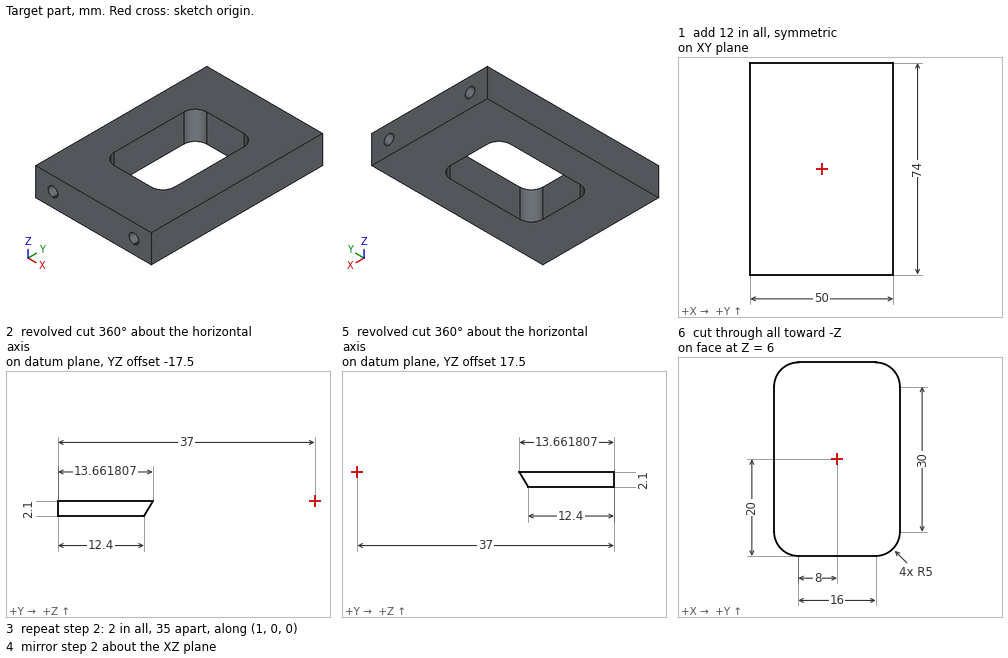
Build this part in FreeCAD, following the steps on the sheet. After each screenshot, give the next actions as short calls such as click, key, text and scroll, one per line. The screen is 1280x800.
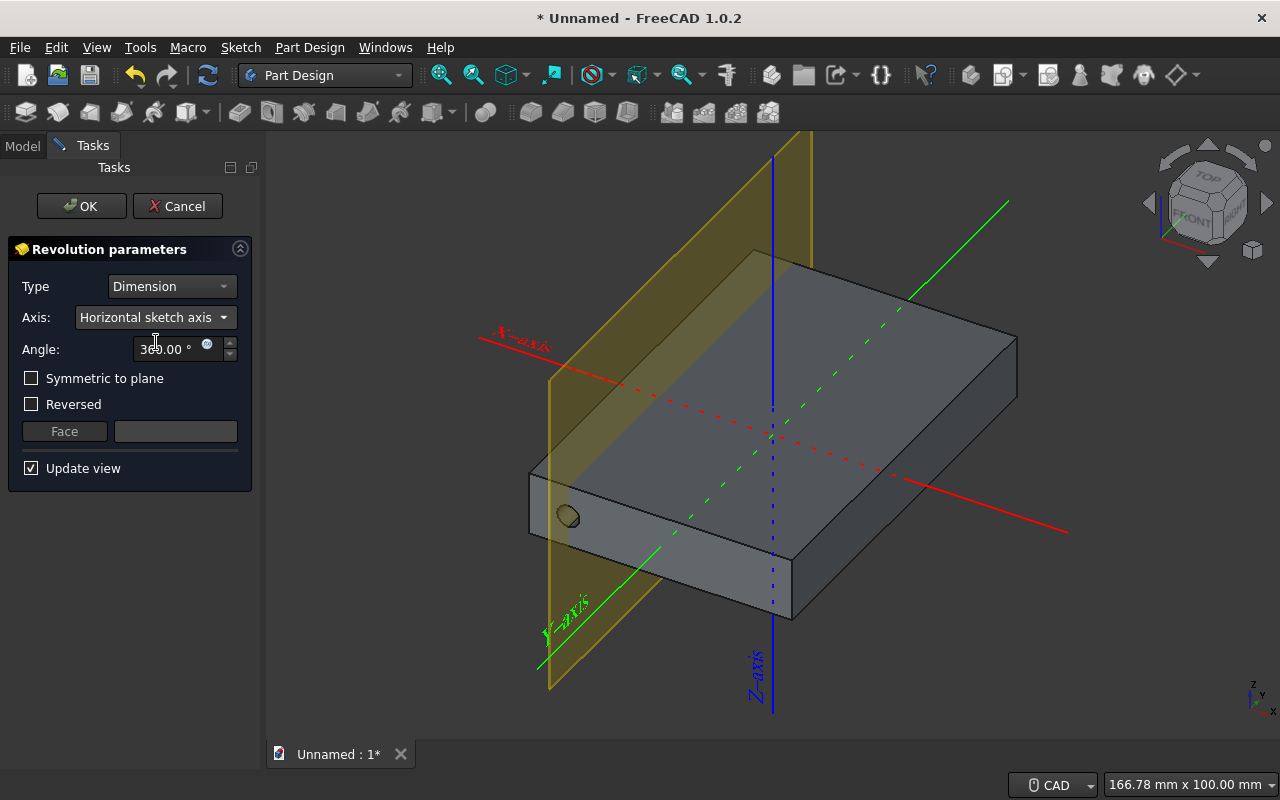
click(82, 206)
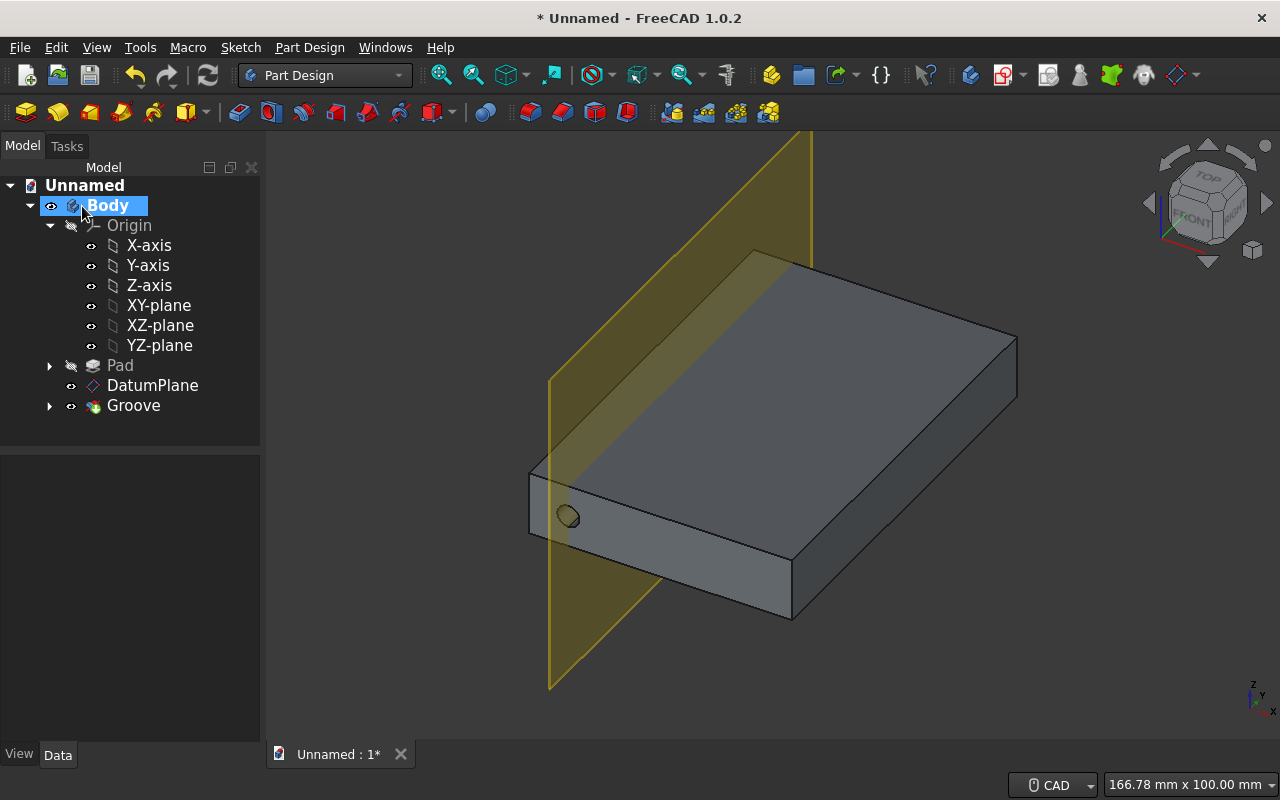
click(116, 386)
key(space)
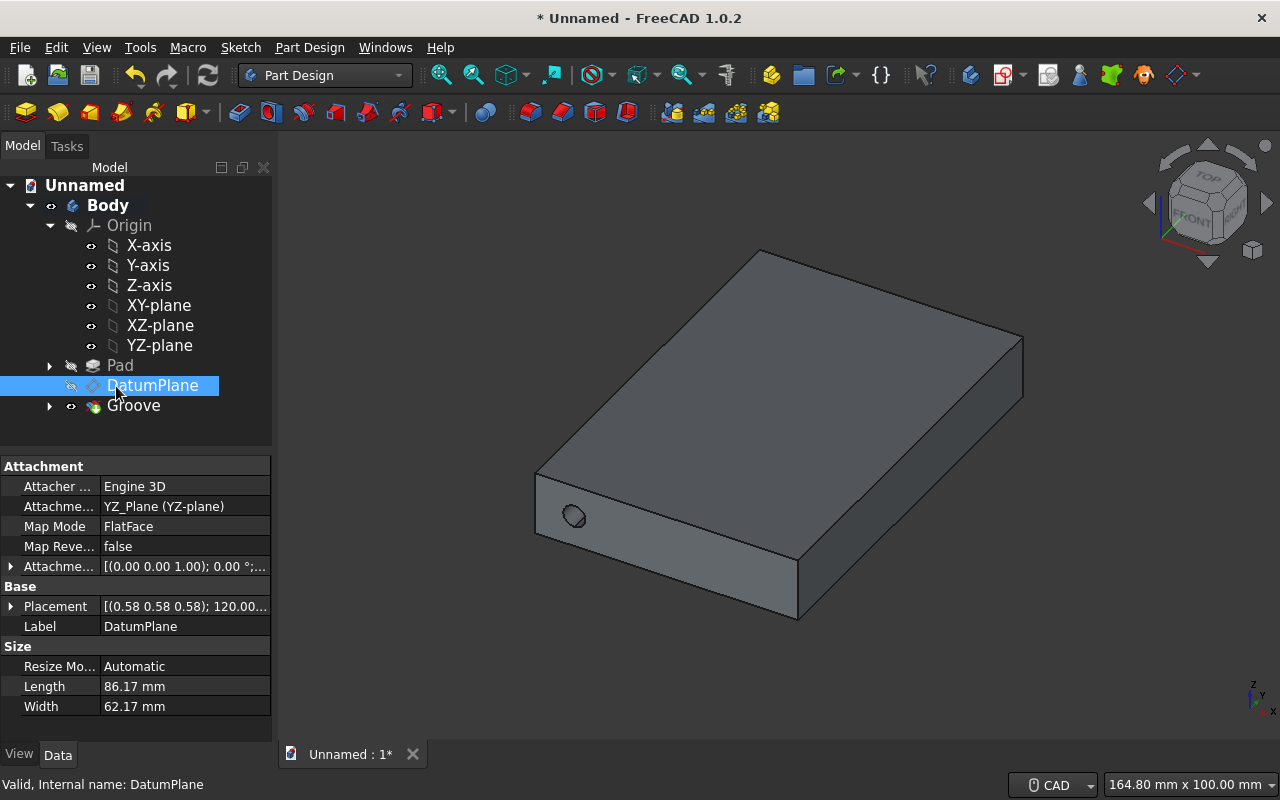
click(116, 406)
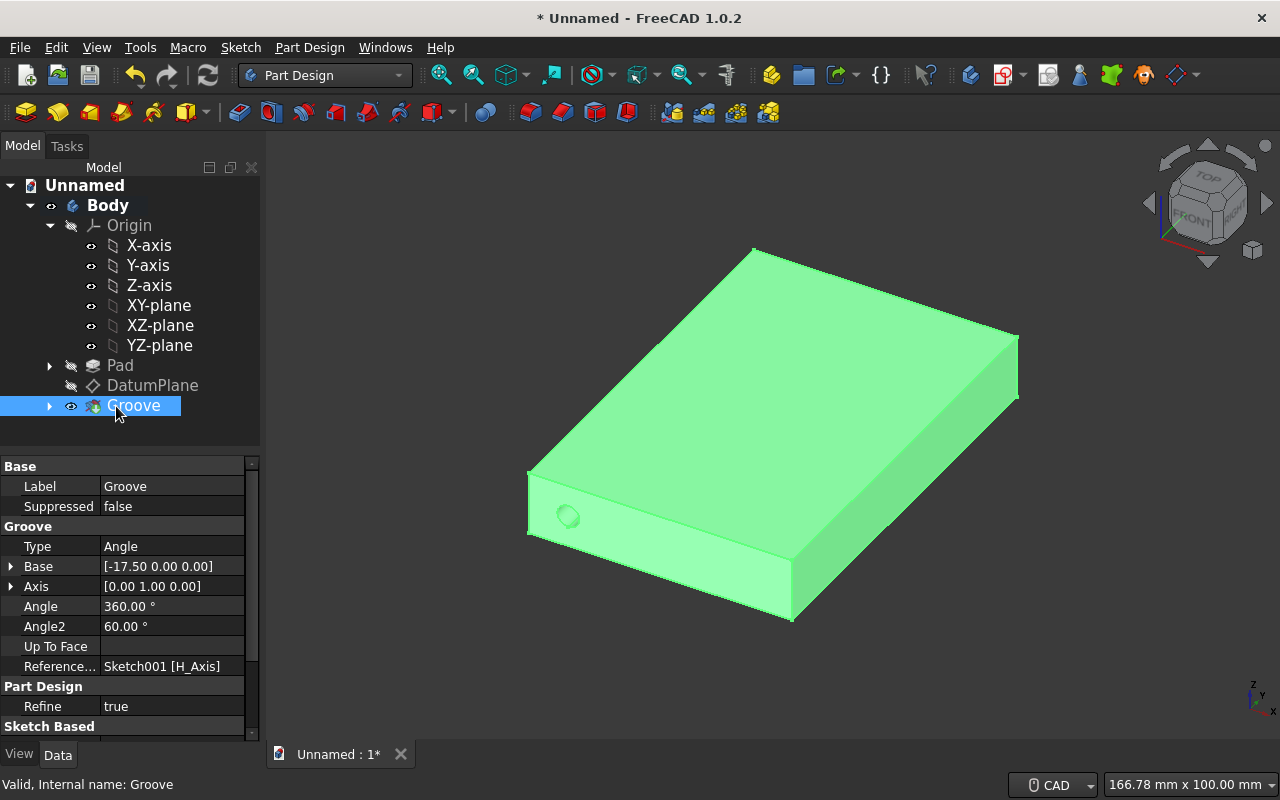
click(704, 112)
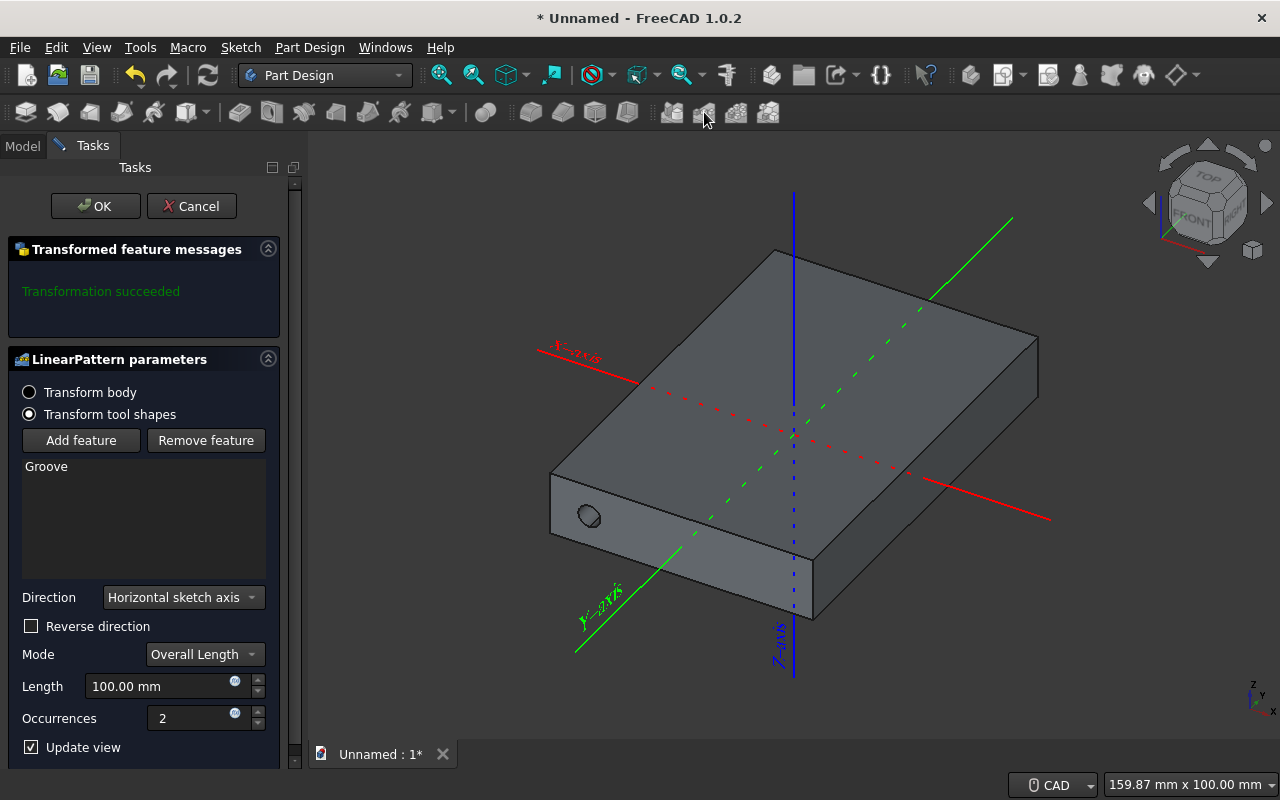
click(184, 598)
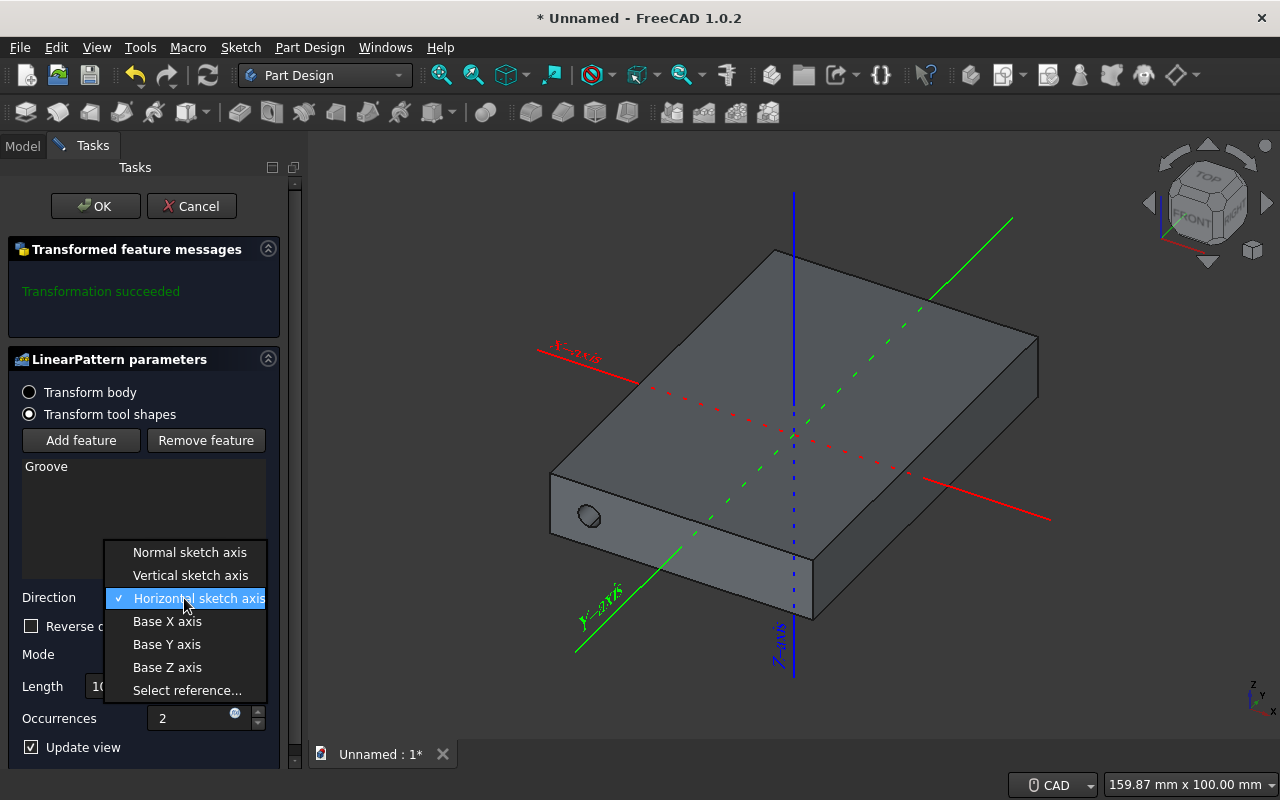
click(184, 622)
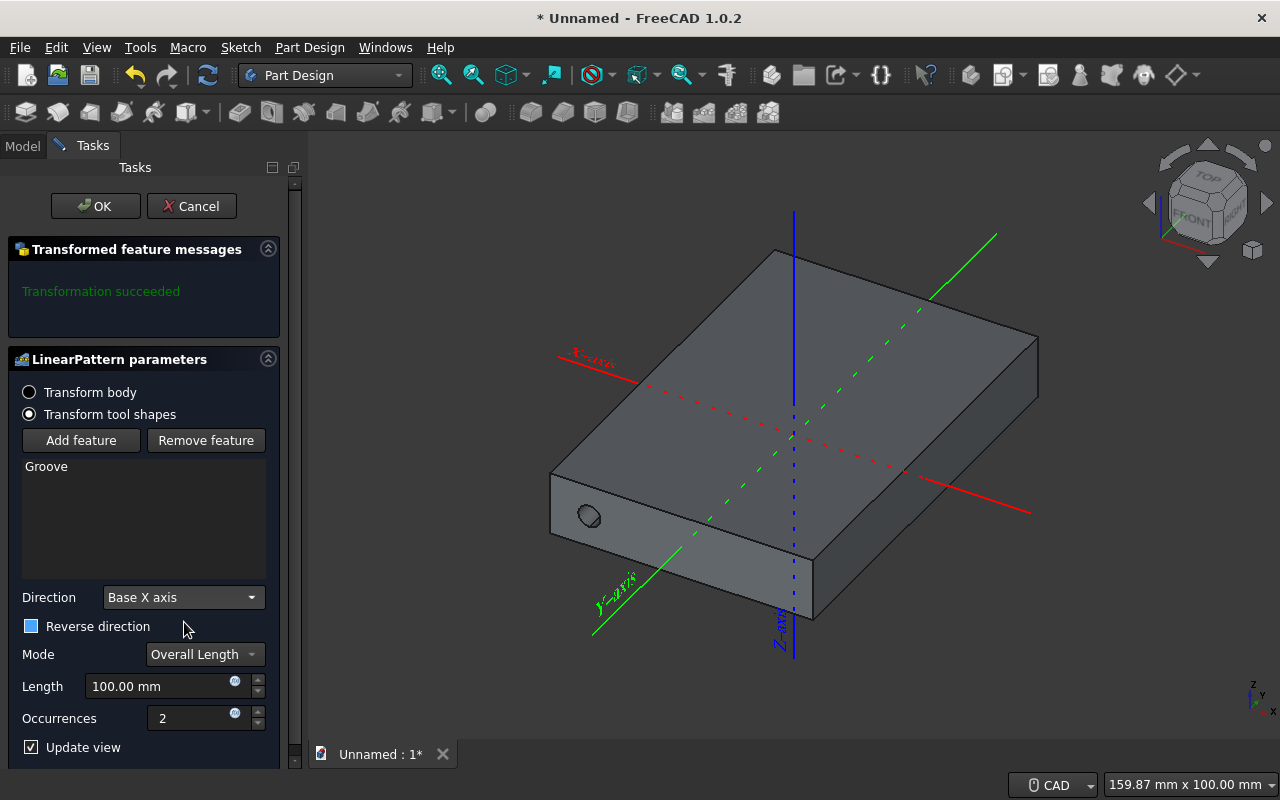
click(206, 654)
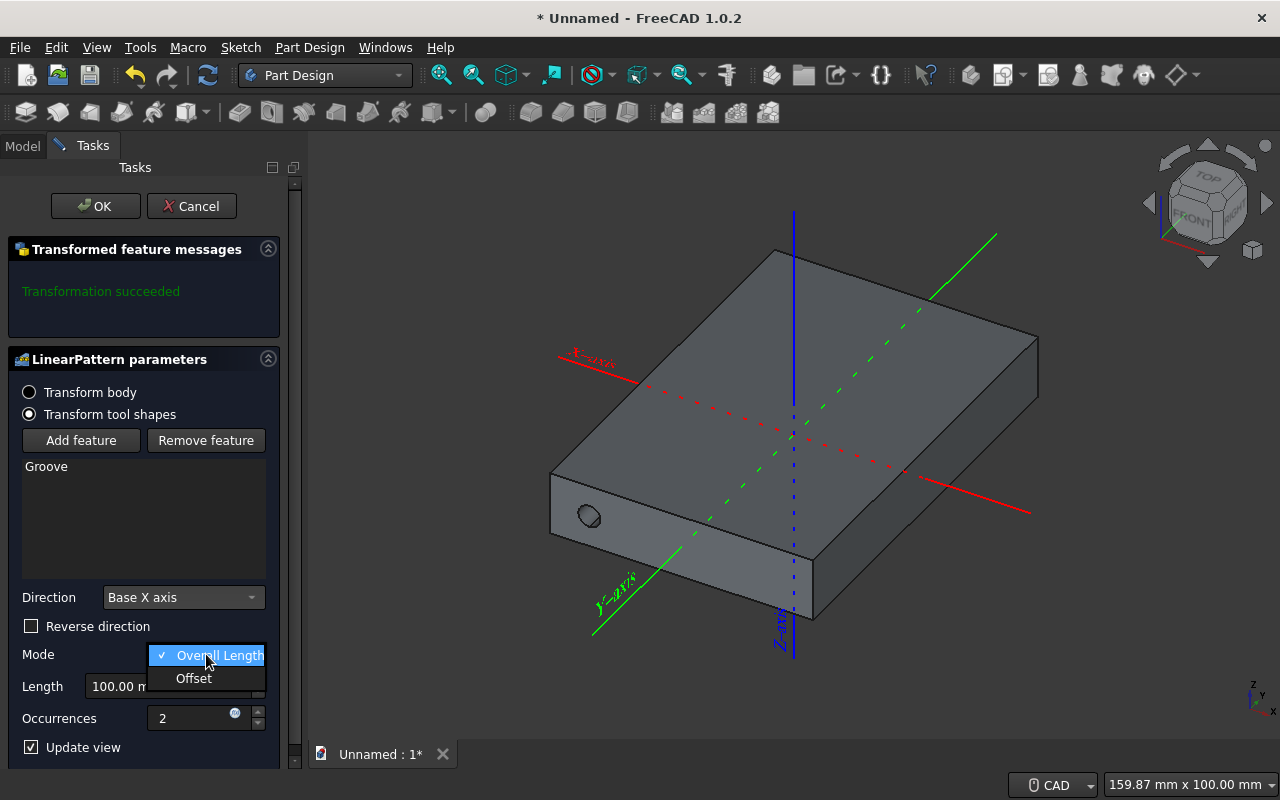
click(206, 678)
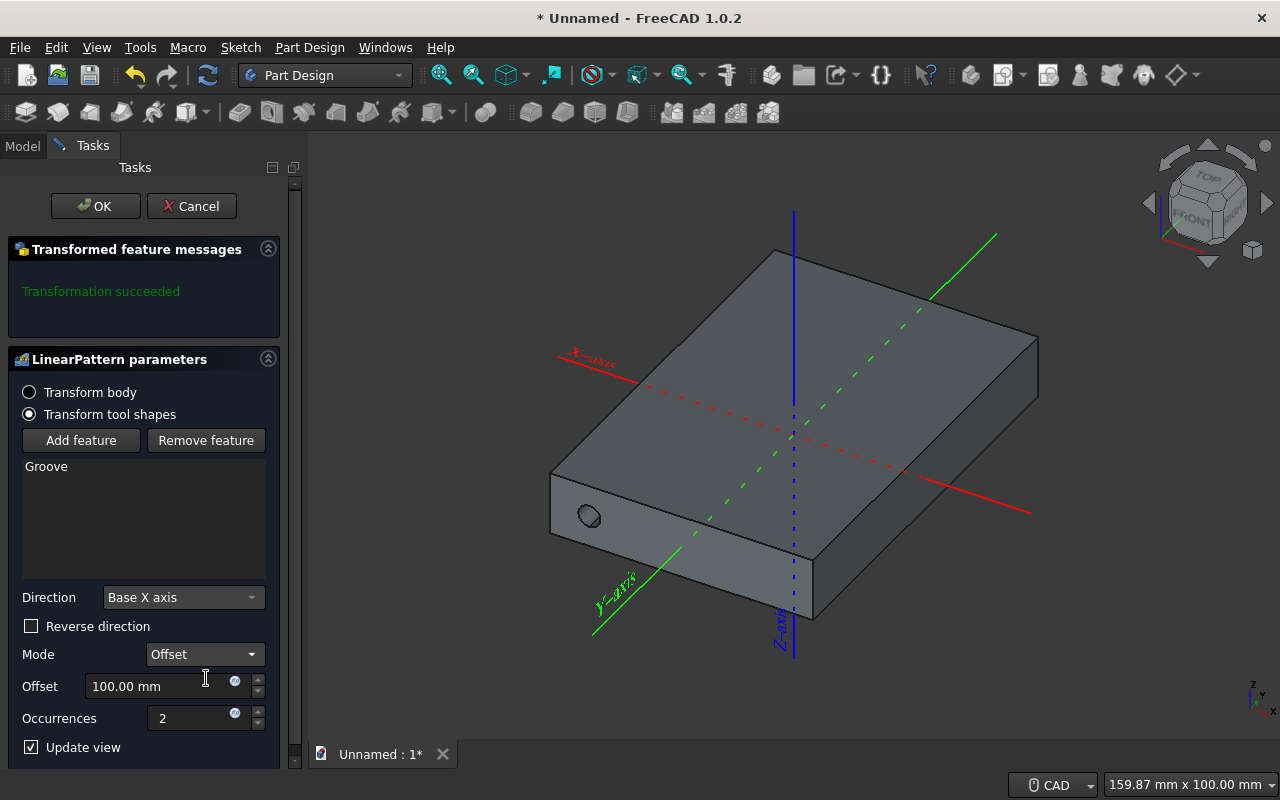
triple_click(168, 686)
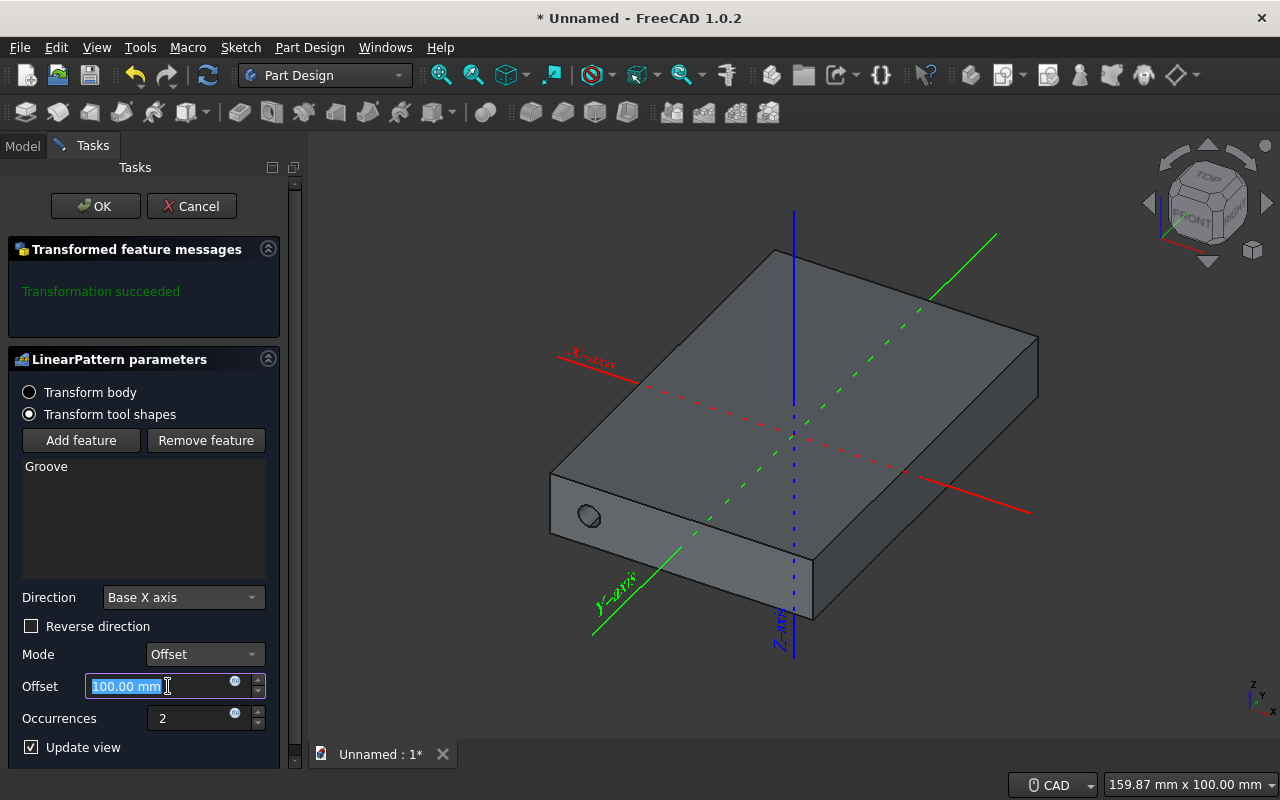
text(35)
key(Tab)